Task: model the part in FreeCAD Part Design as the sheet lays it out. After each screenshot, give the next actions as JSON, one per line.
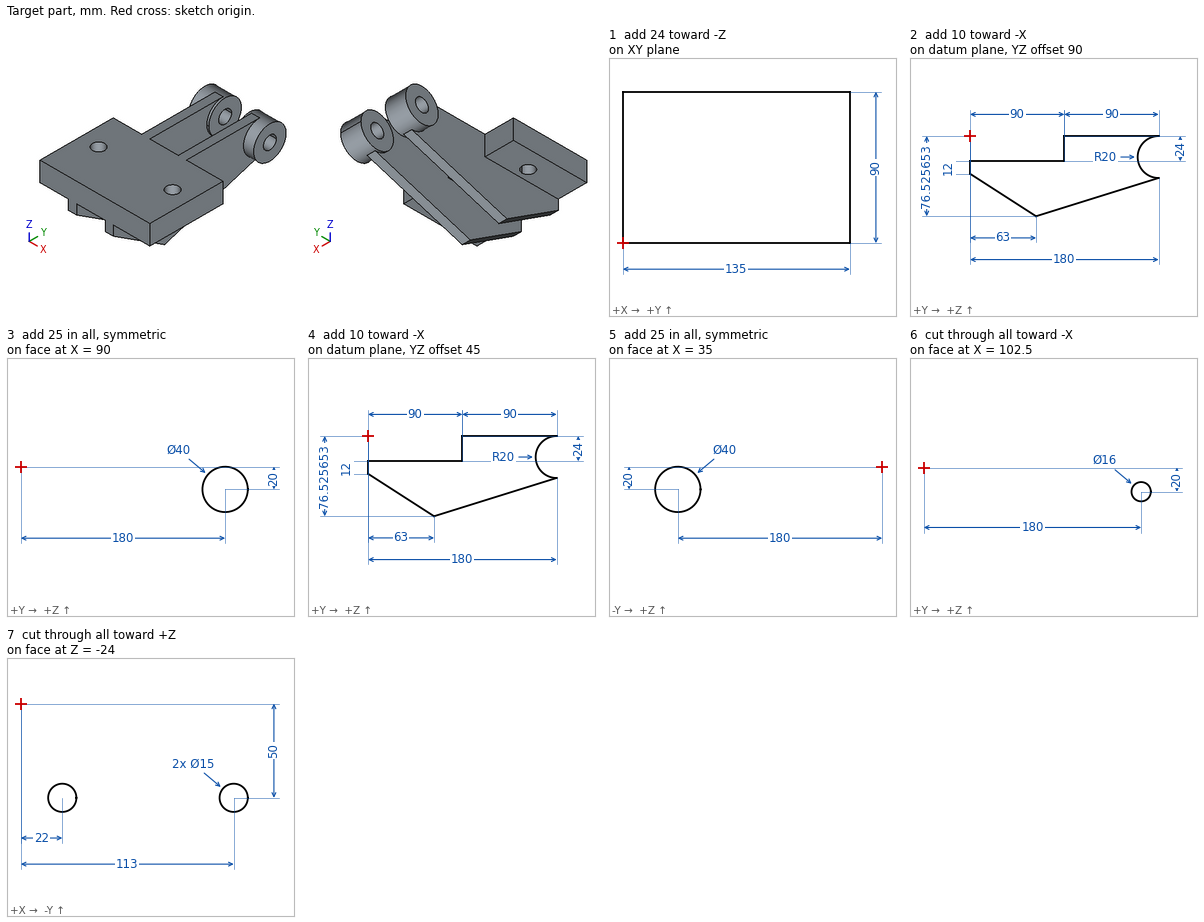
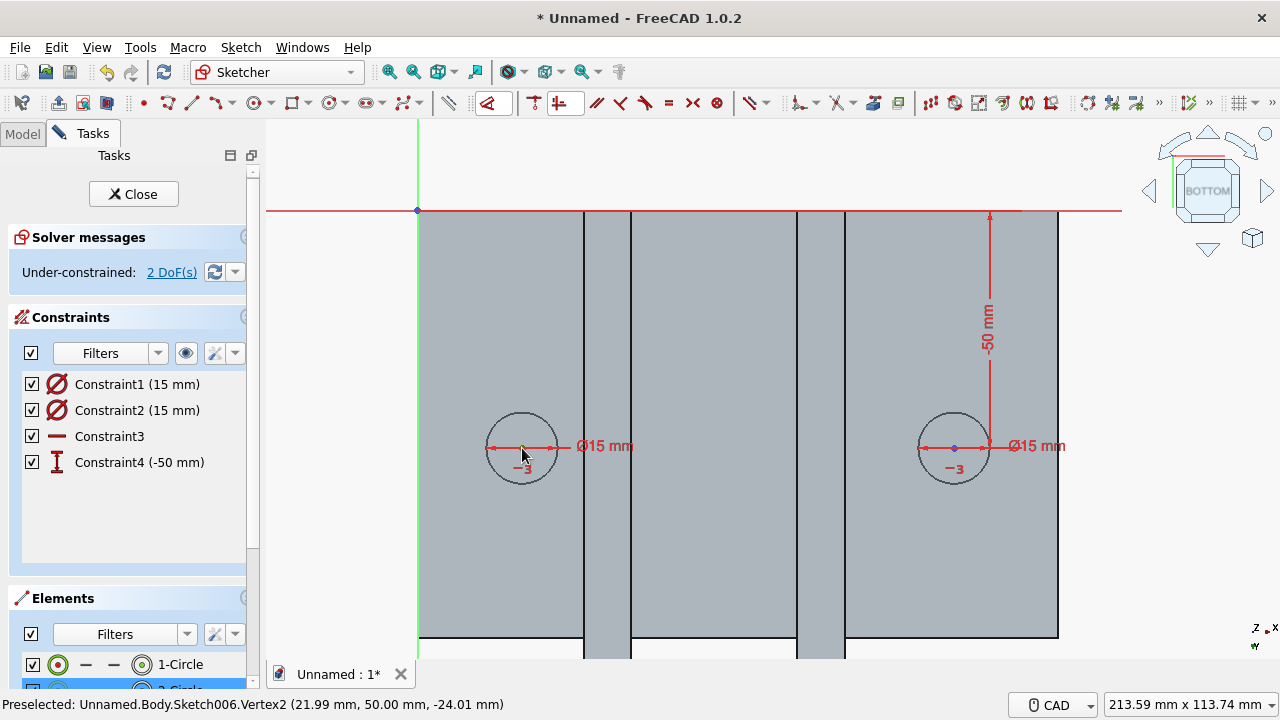
{"action": "left_click", "coordinate": [506, 104]}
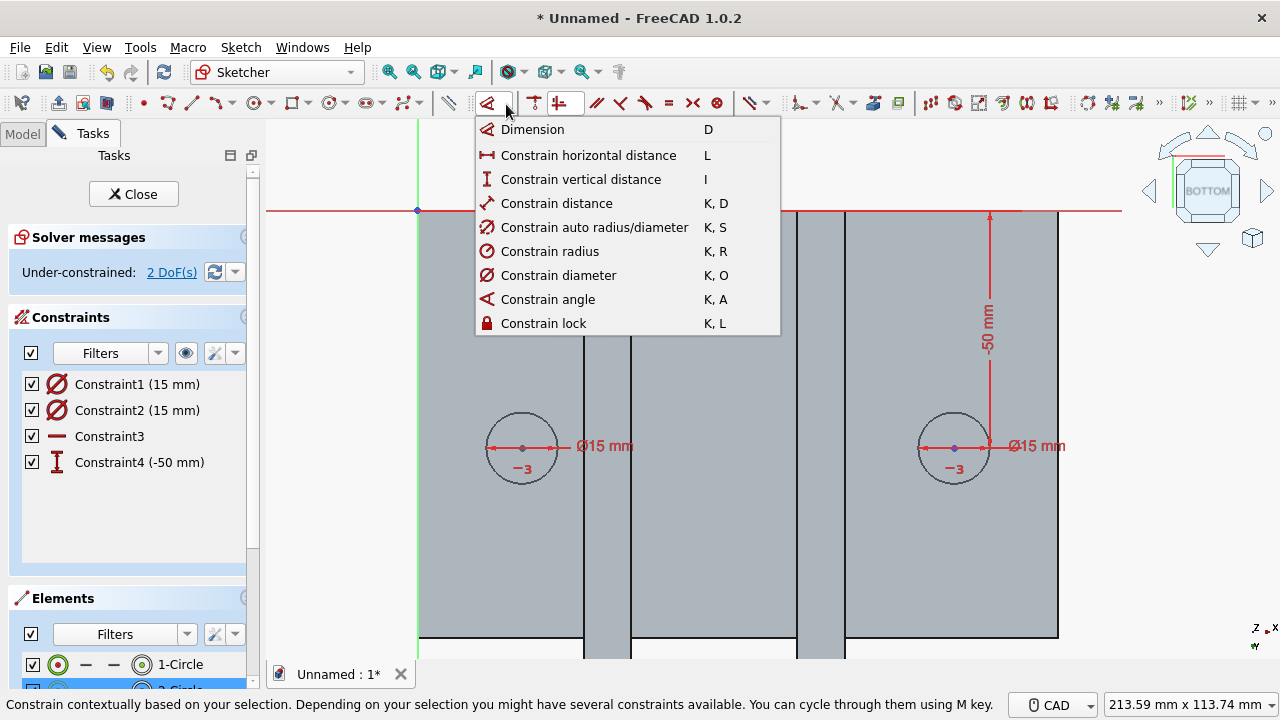
{"action": "left_click", "coordinate": [628, 155]}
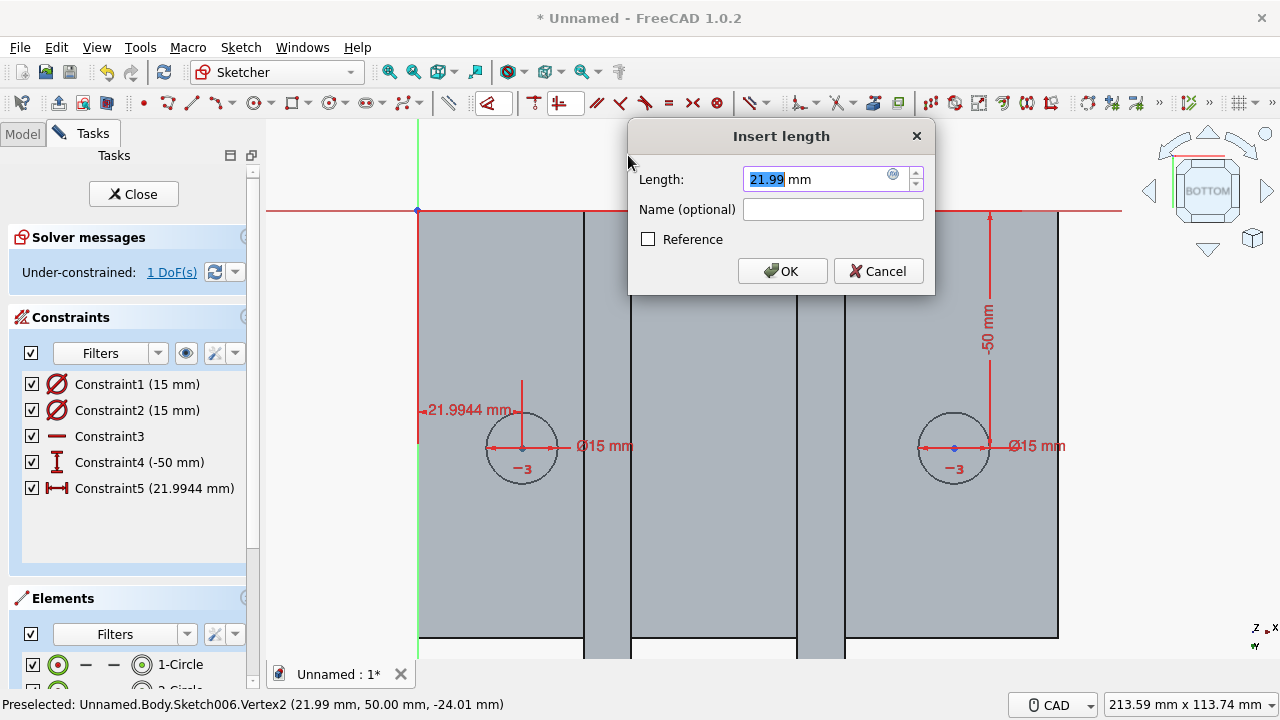
{"action": "type", "text": "22"}
{"action": "key", "text": "Return"}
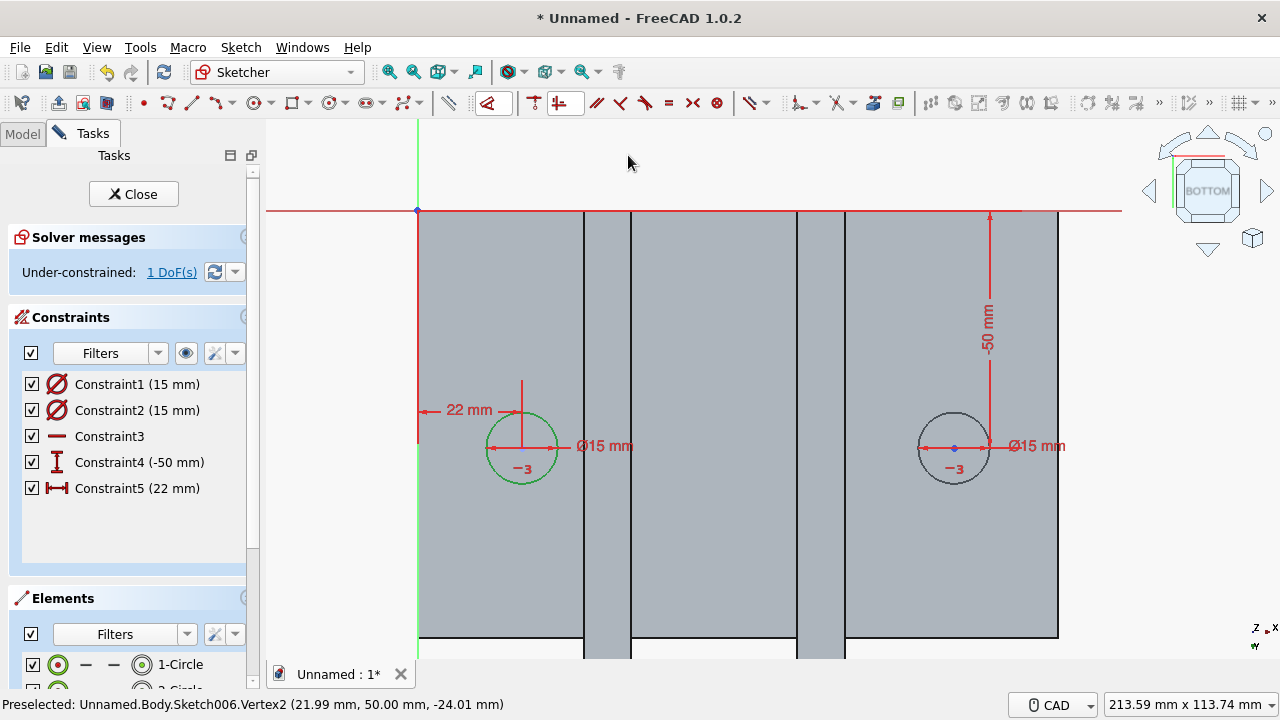
{"action": "left_click", "coordinate": [954, 448]}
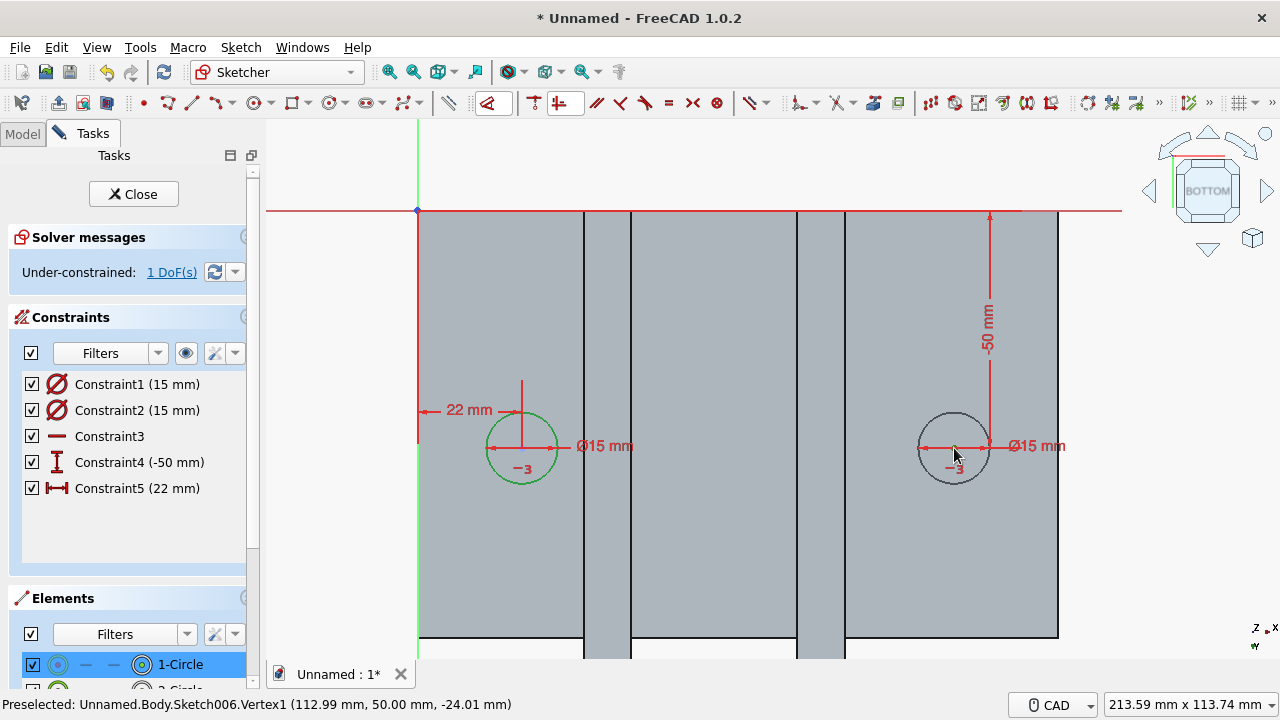
{"action": "left_click", "coordinate": [506, 104]}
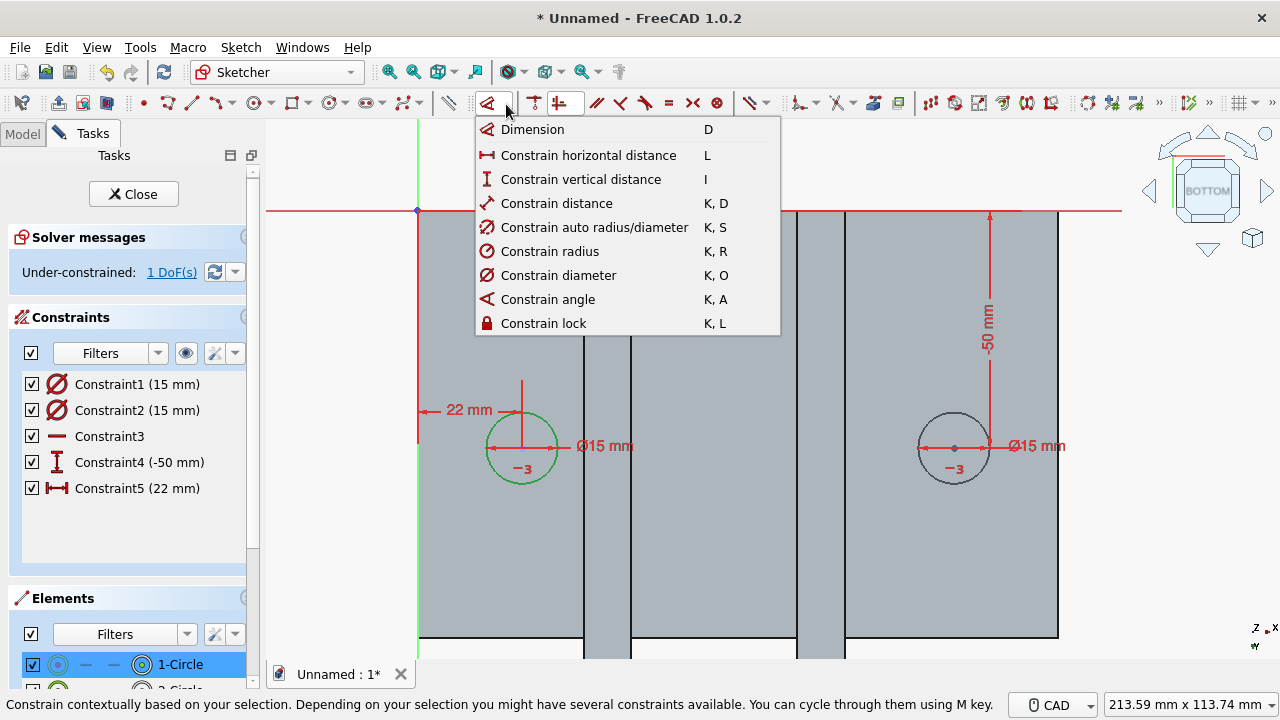
{"action": "left_click", "coordinate": [628, 155]}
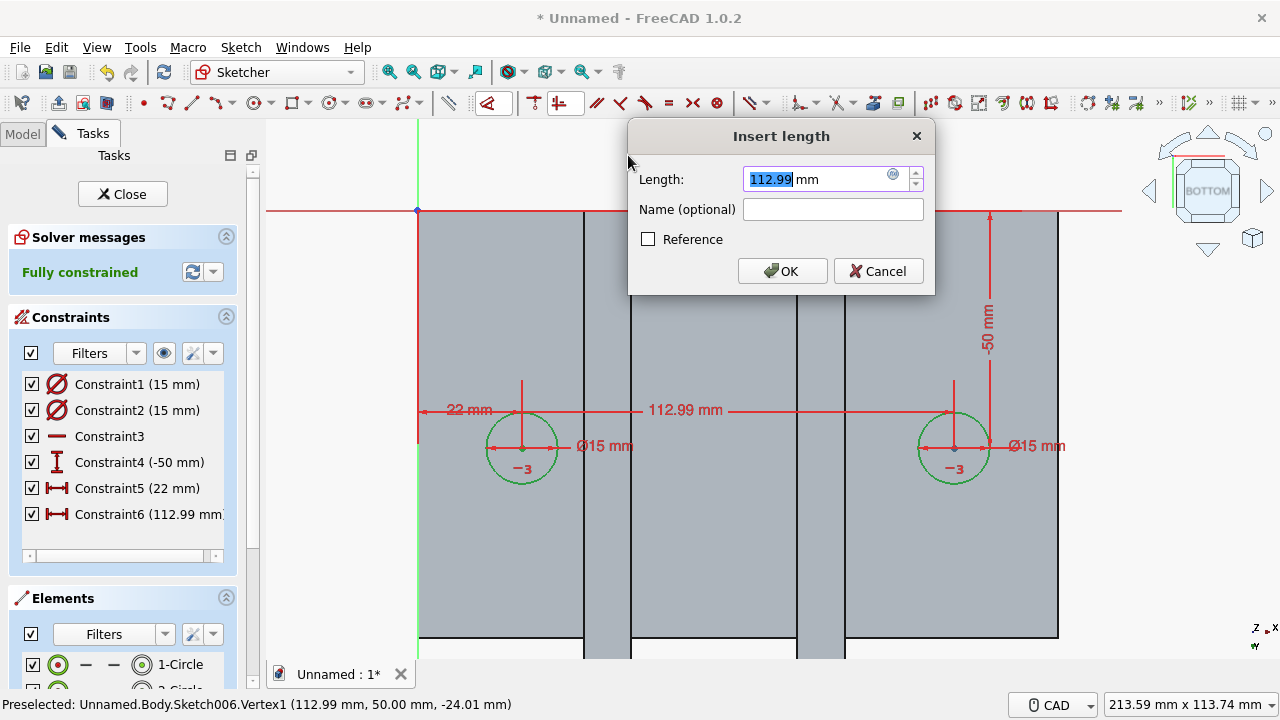
{"action": "type", "text": "113"}
{"action": "key", "text": "Return"}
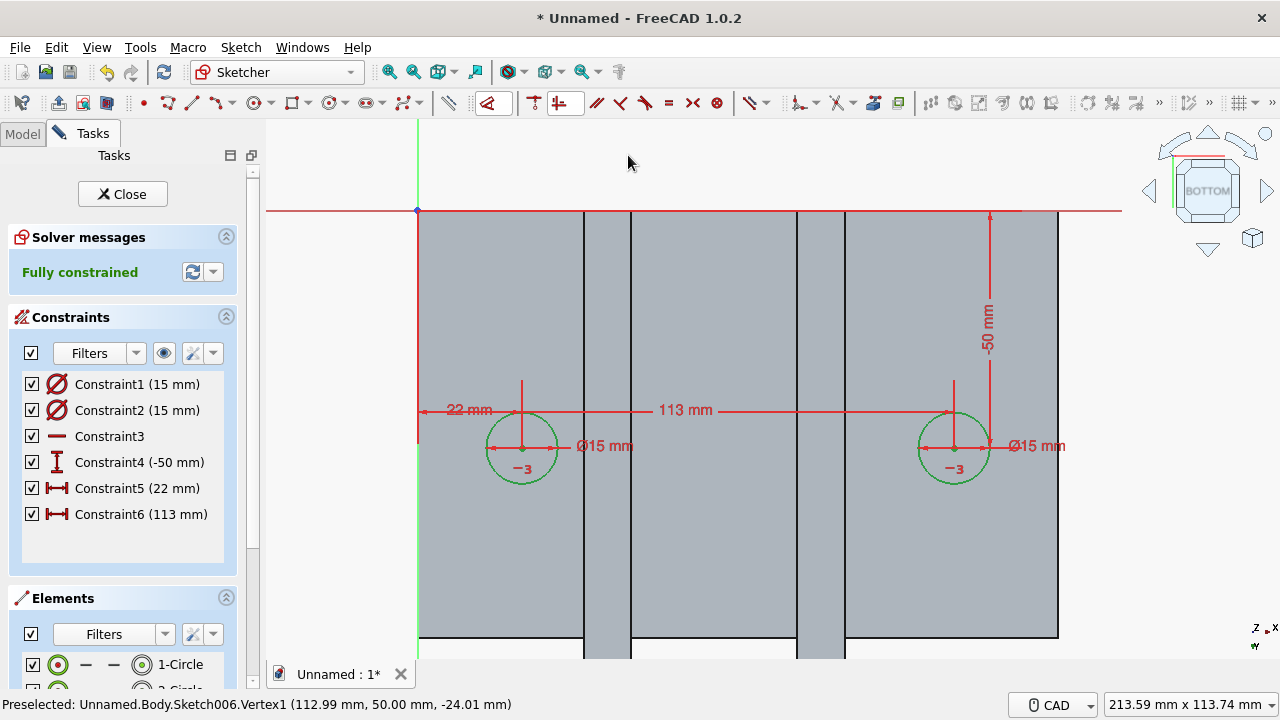
{"action": "left_click", "coordinate": [123, 194]}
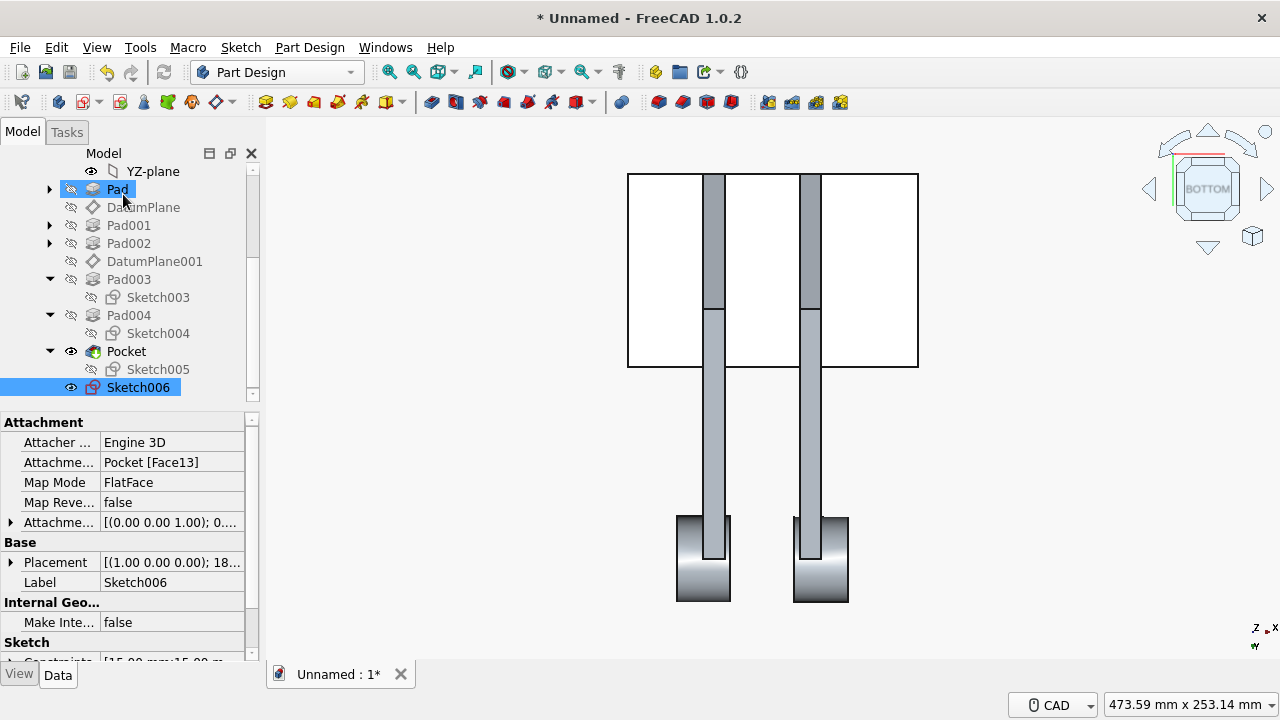
{"action": "left_click", "coordinate": [432, 102]}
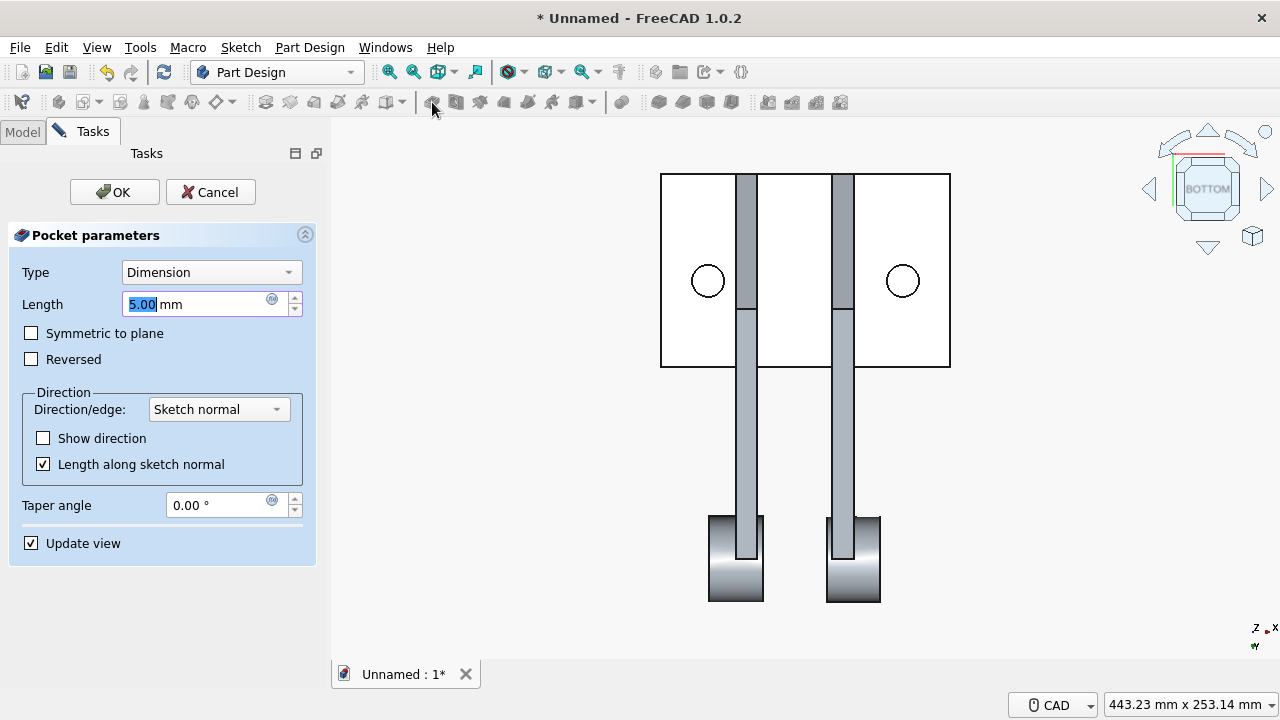
{"action": "left_click", "coordinate": [212, 272]}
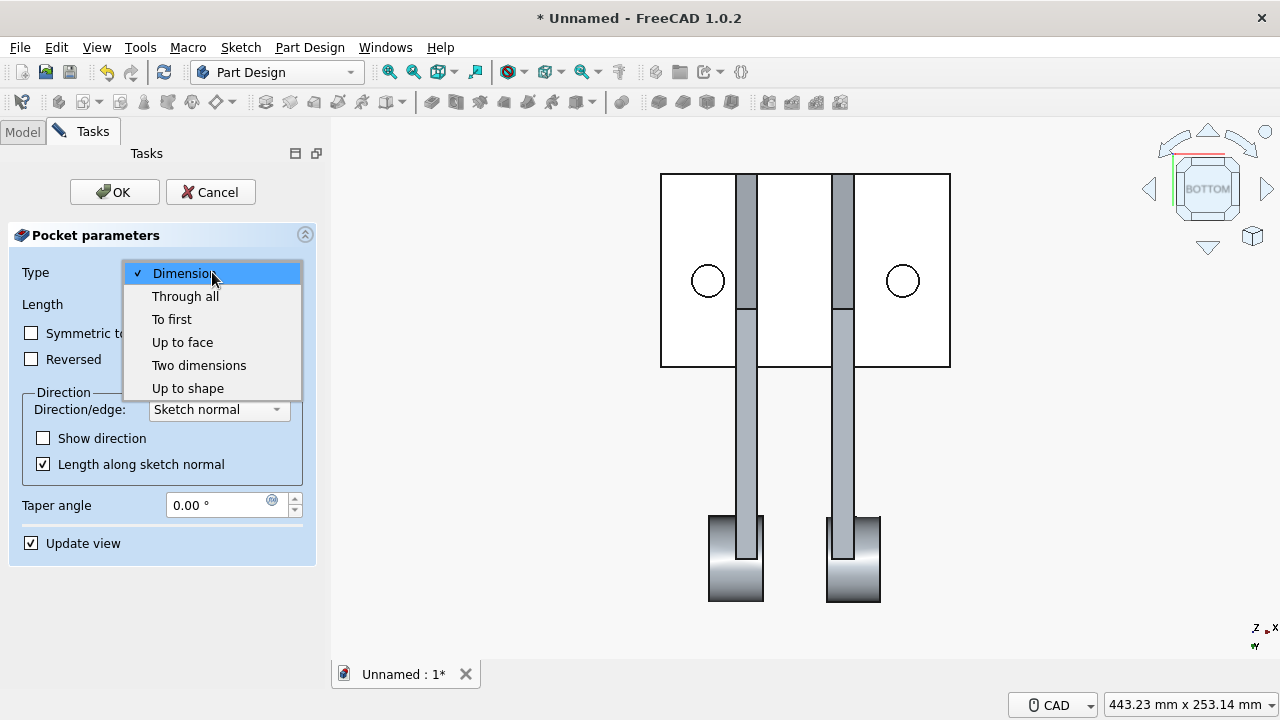
{"action": "left_click", "coordinate": [212, 296]}